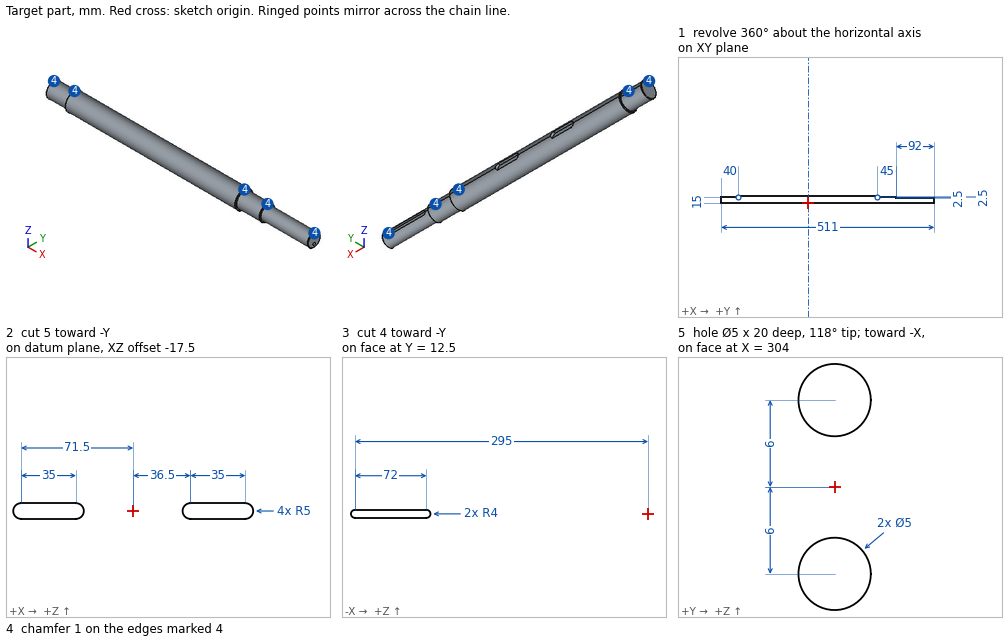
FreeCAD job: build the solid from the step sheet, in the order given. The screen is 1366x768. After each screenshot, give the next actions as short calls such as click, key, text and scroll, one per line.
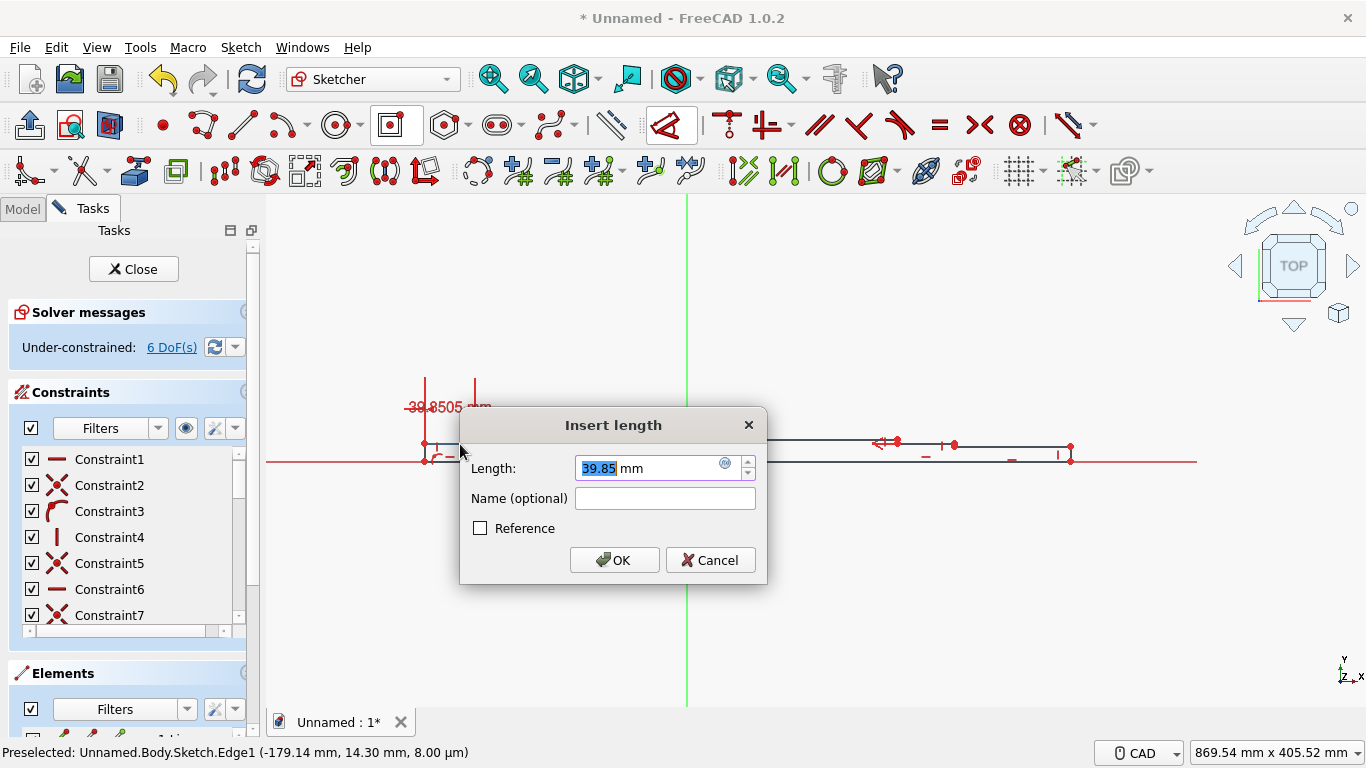
text(40)
key(Return)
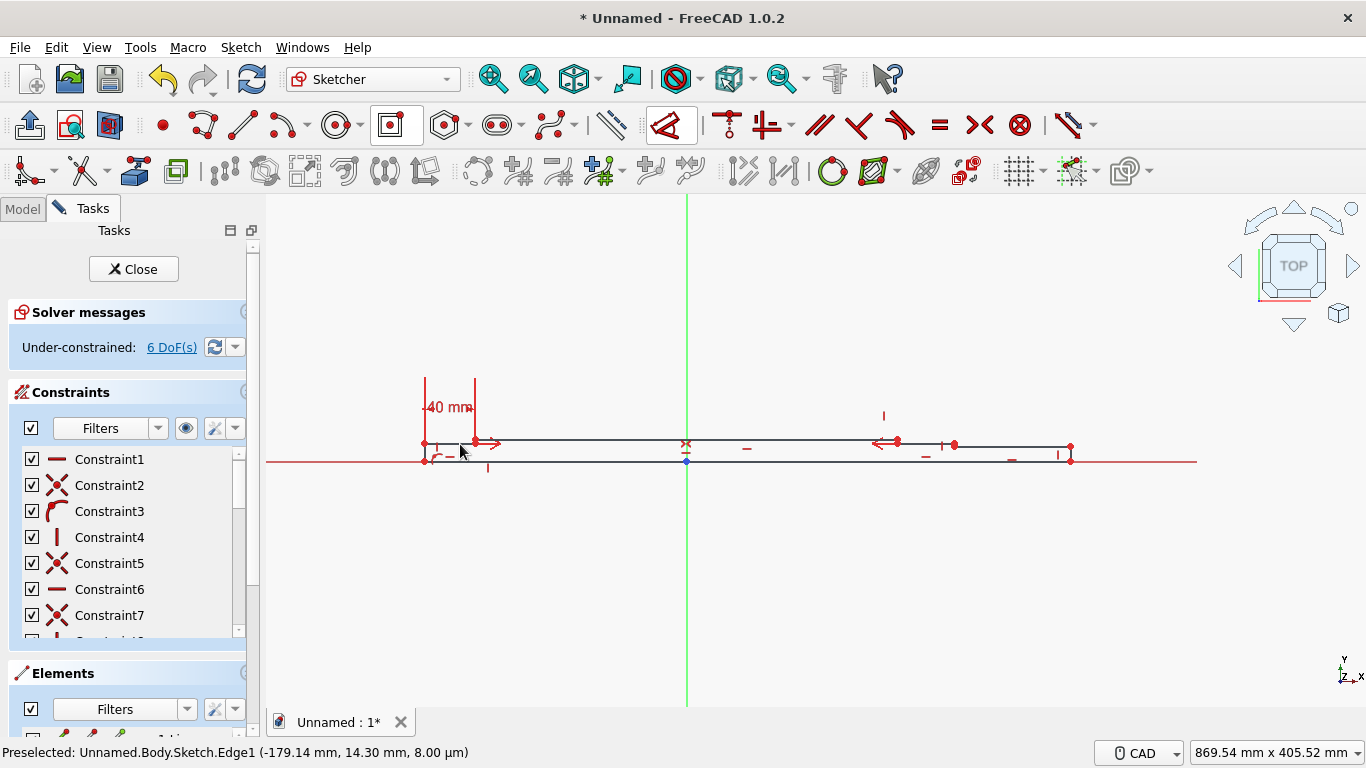
scroll(425, 453, up, 4)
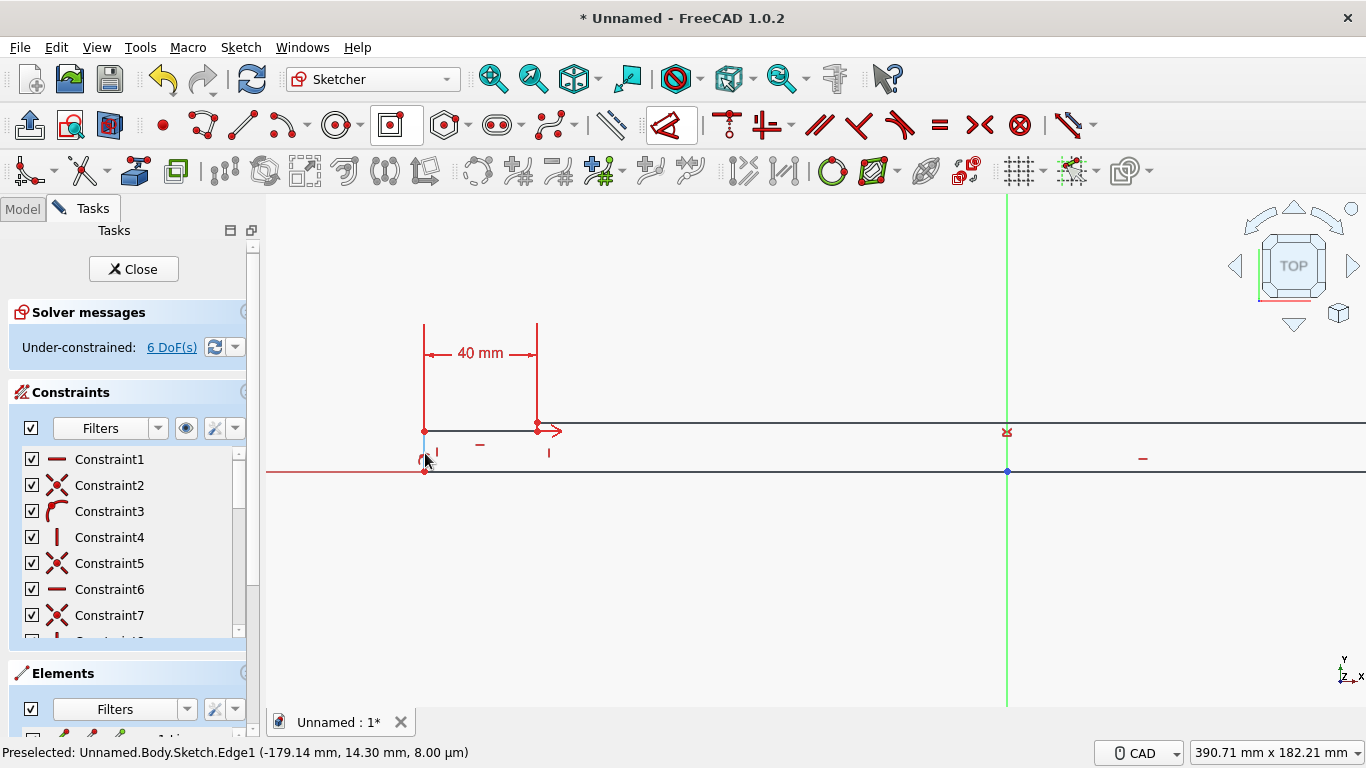
click(424, 451)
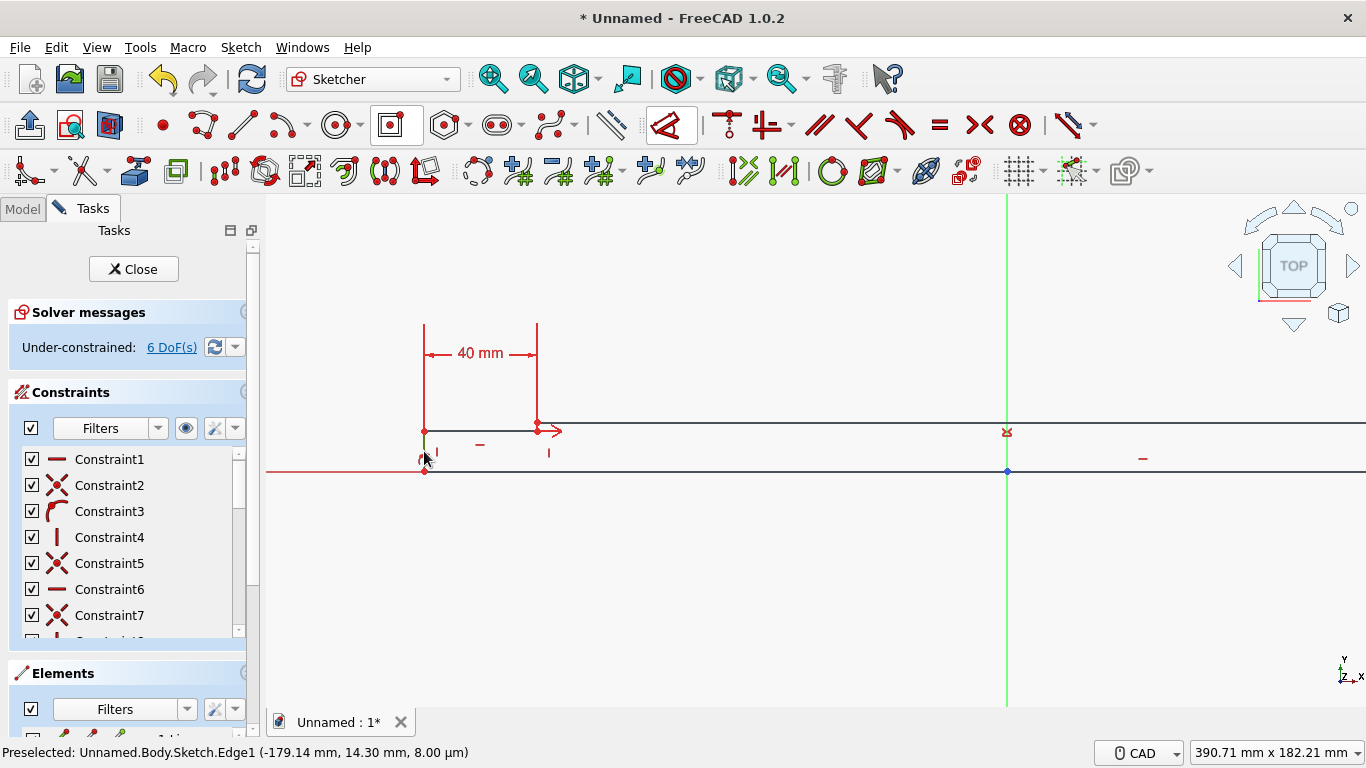
click(692, 126)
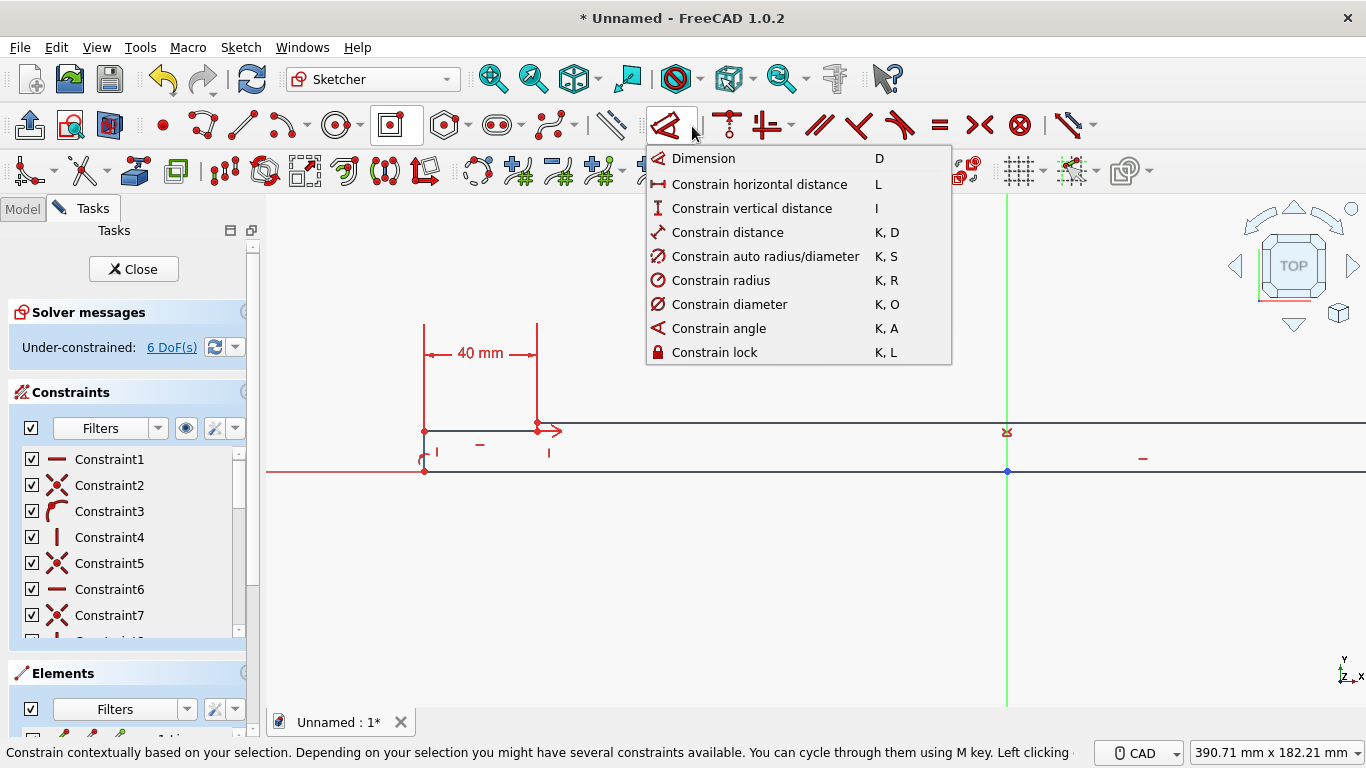
click(799, 208)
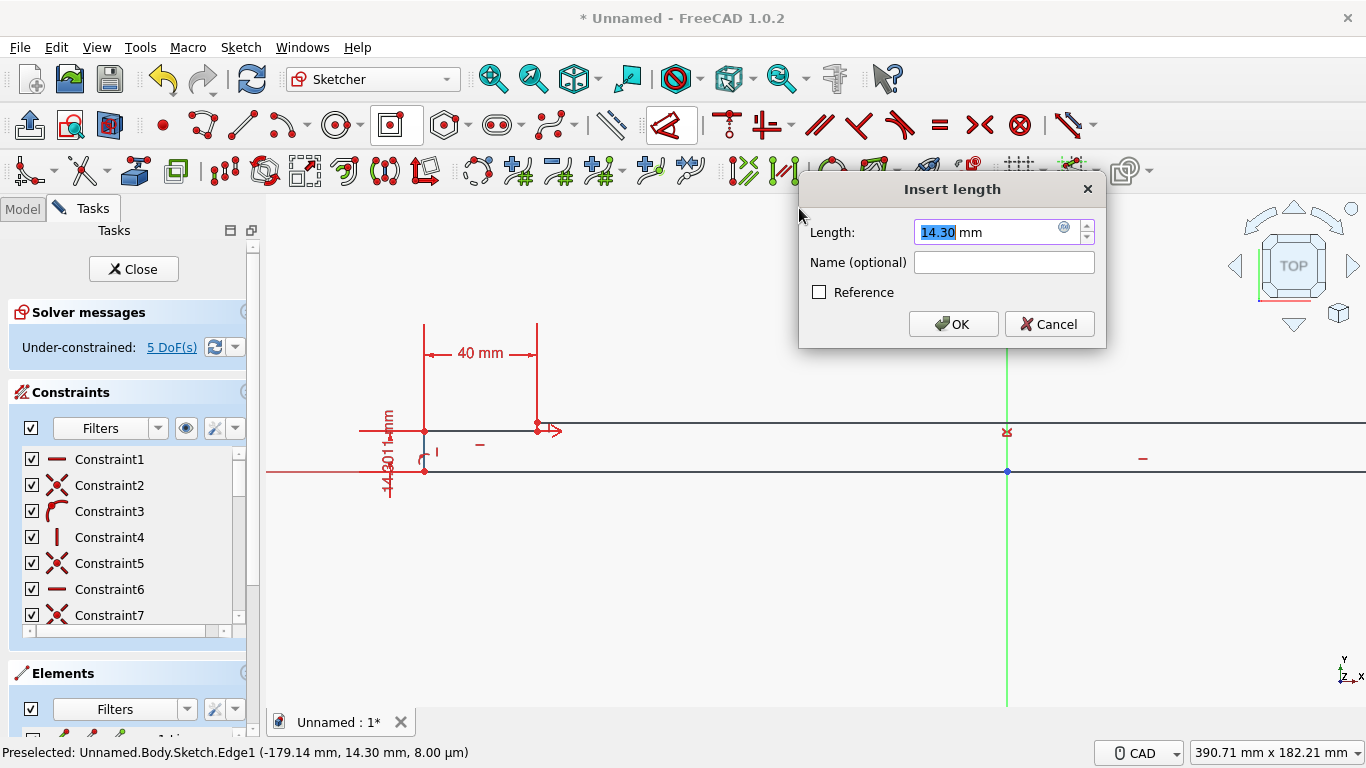
text(15)
key(Return)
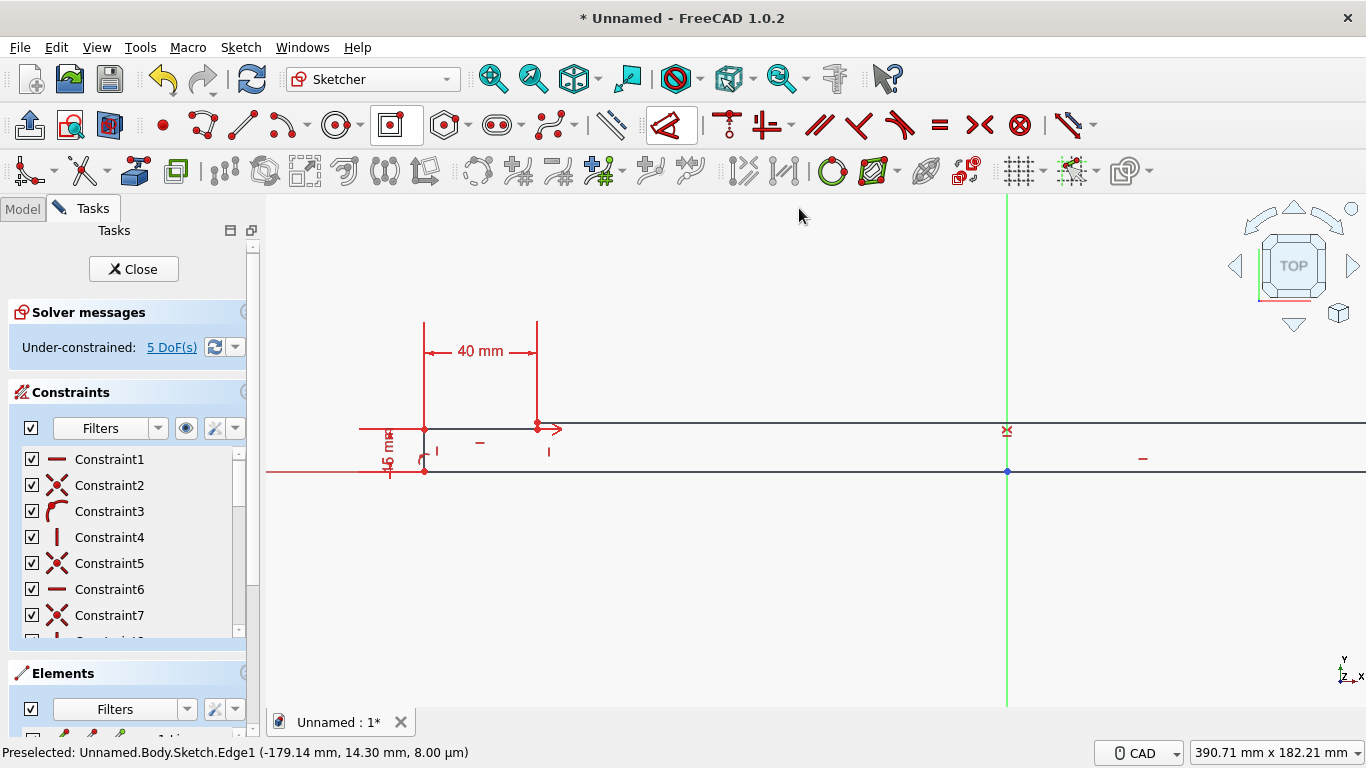
scroll(424, 453, down, 4)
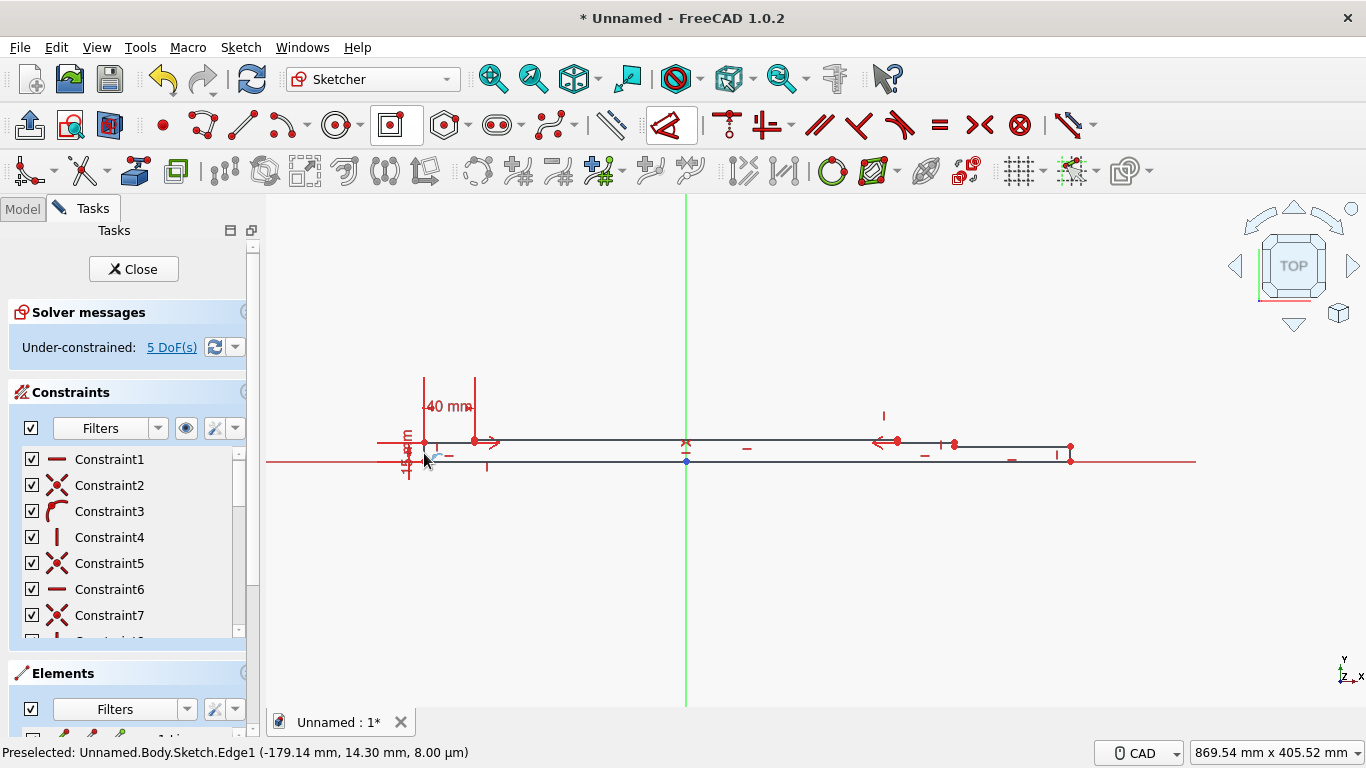
click(1036, 447)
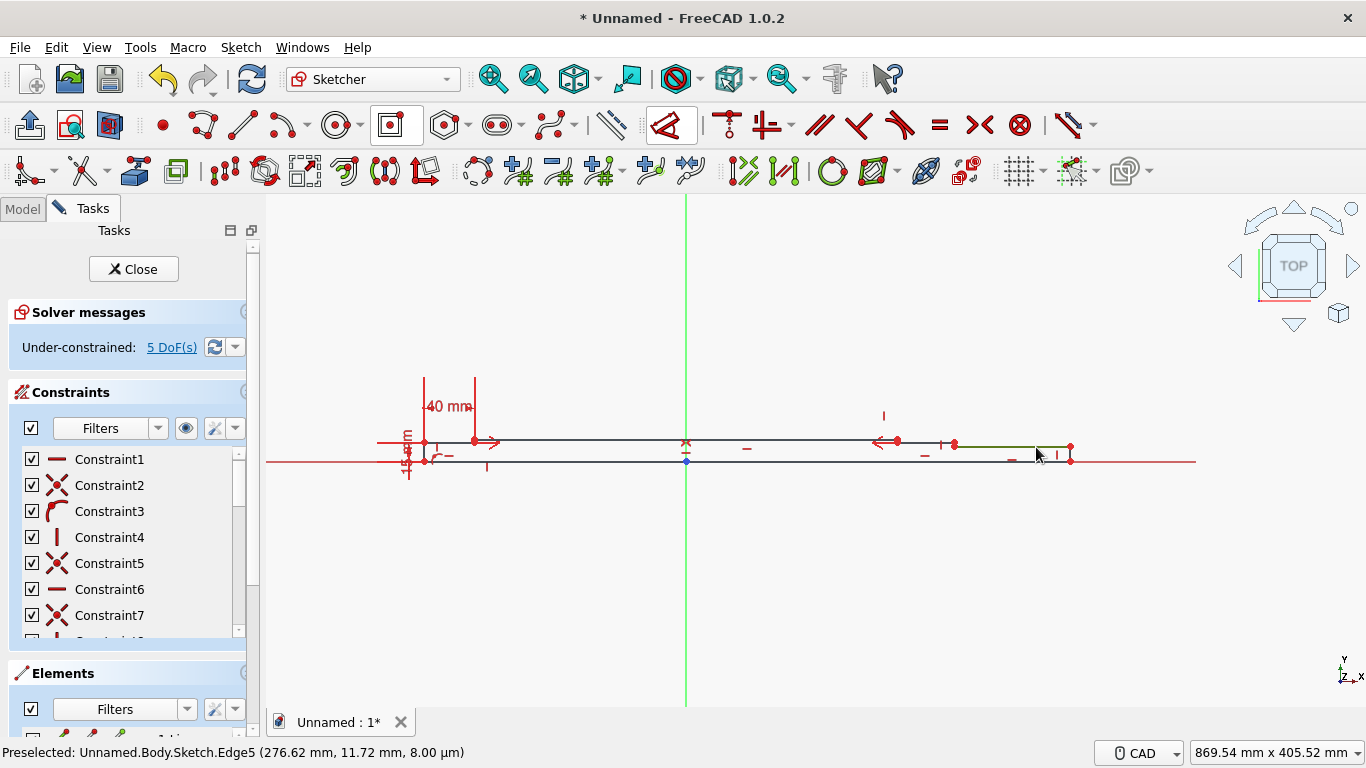
click(692, 126)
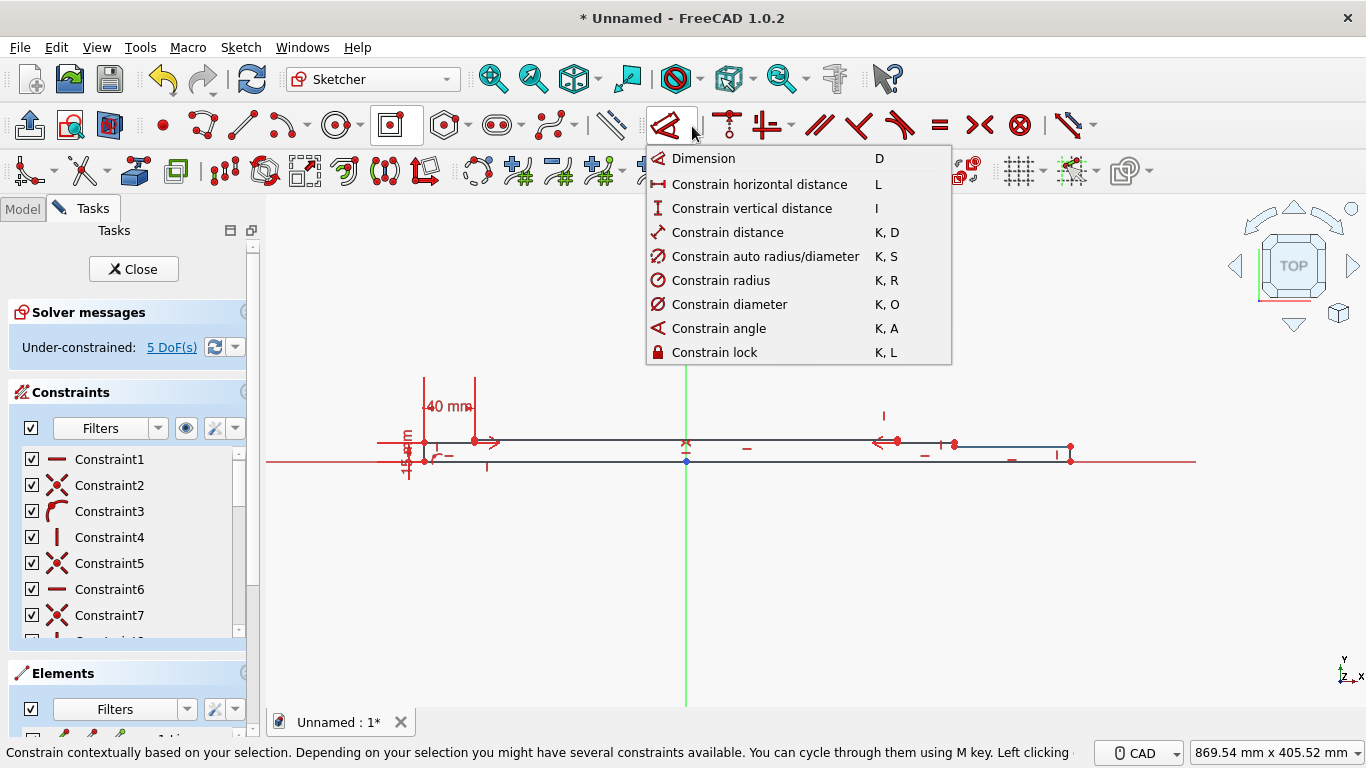
click(799, 184)